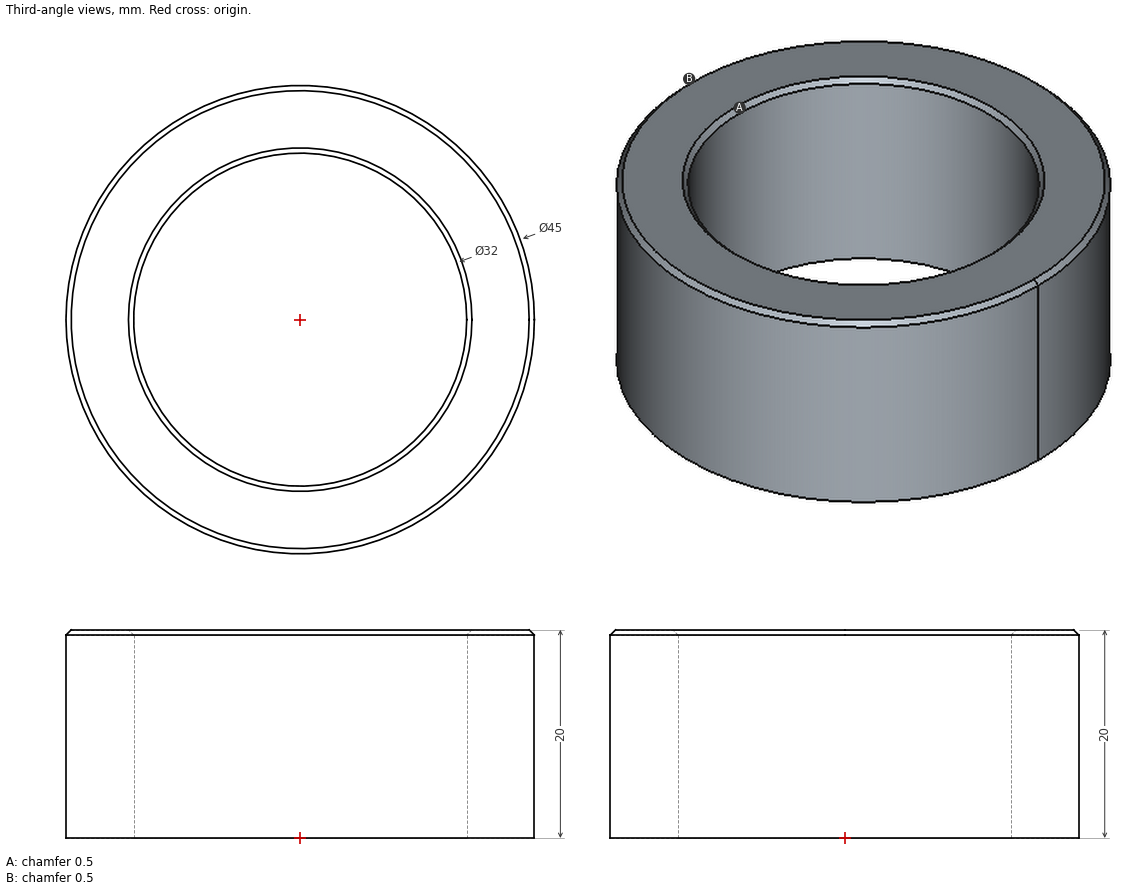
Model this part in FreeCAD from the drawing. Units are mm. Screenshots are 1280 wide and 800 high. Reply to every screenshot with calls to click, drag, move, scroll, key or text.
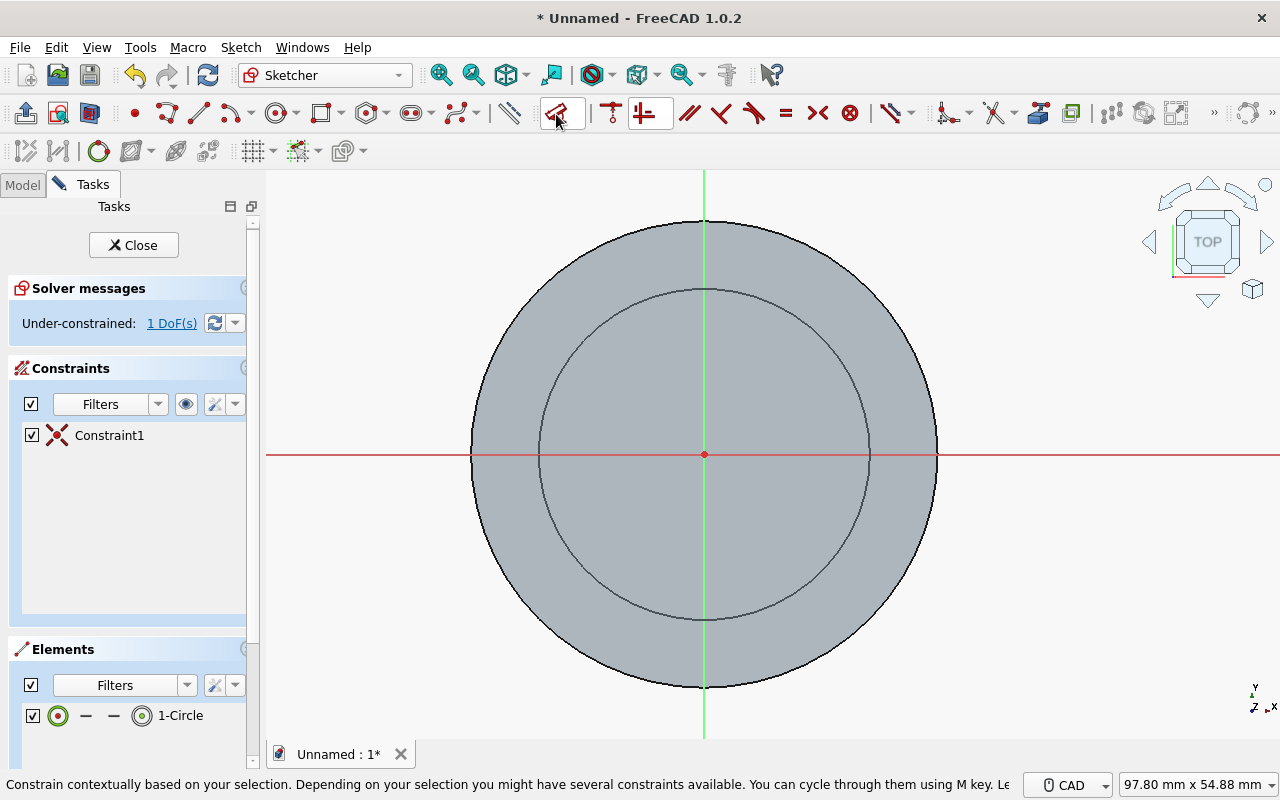
click(821, 337)
click(844, 314)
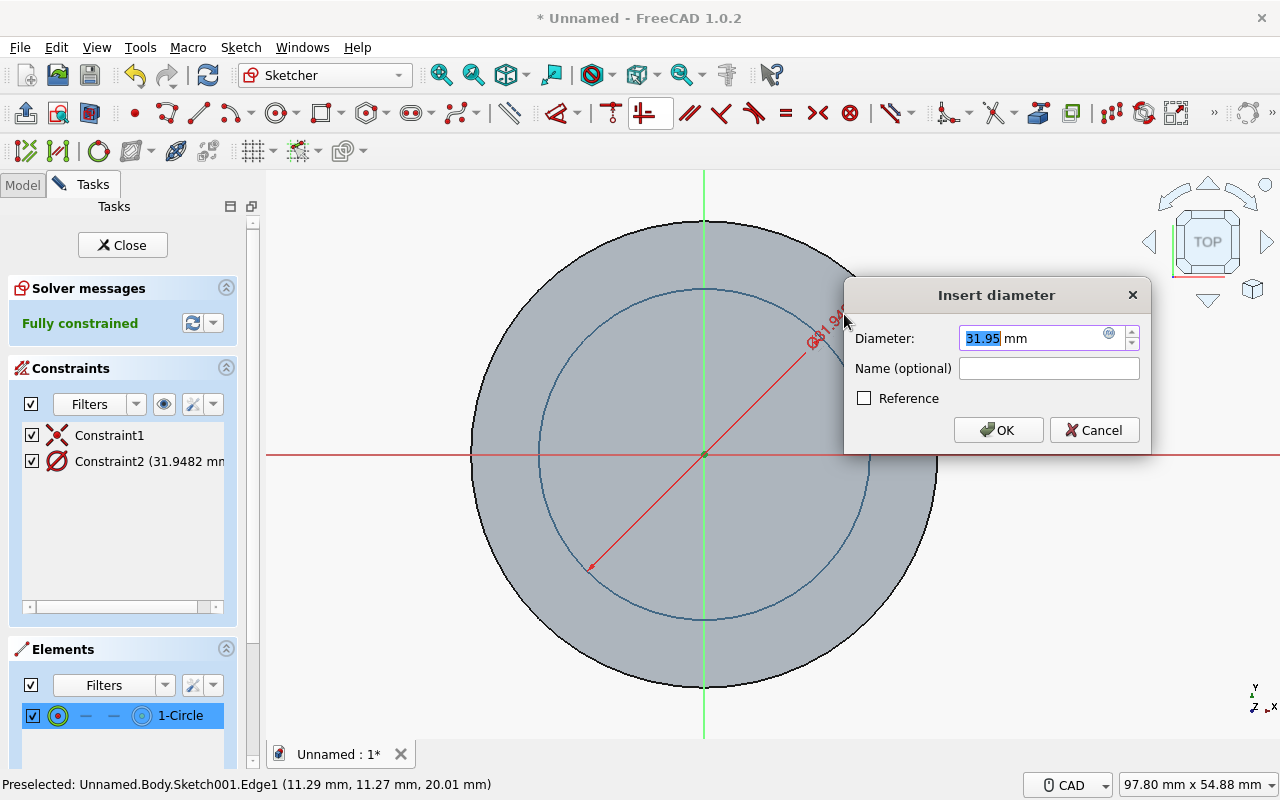
text(32)
key(Return)
key(Escape)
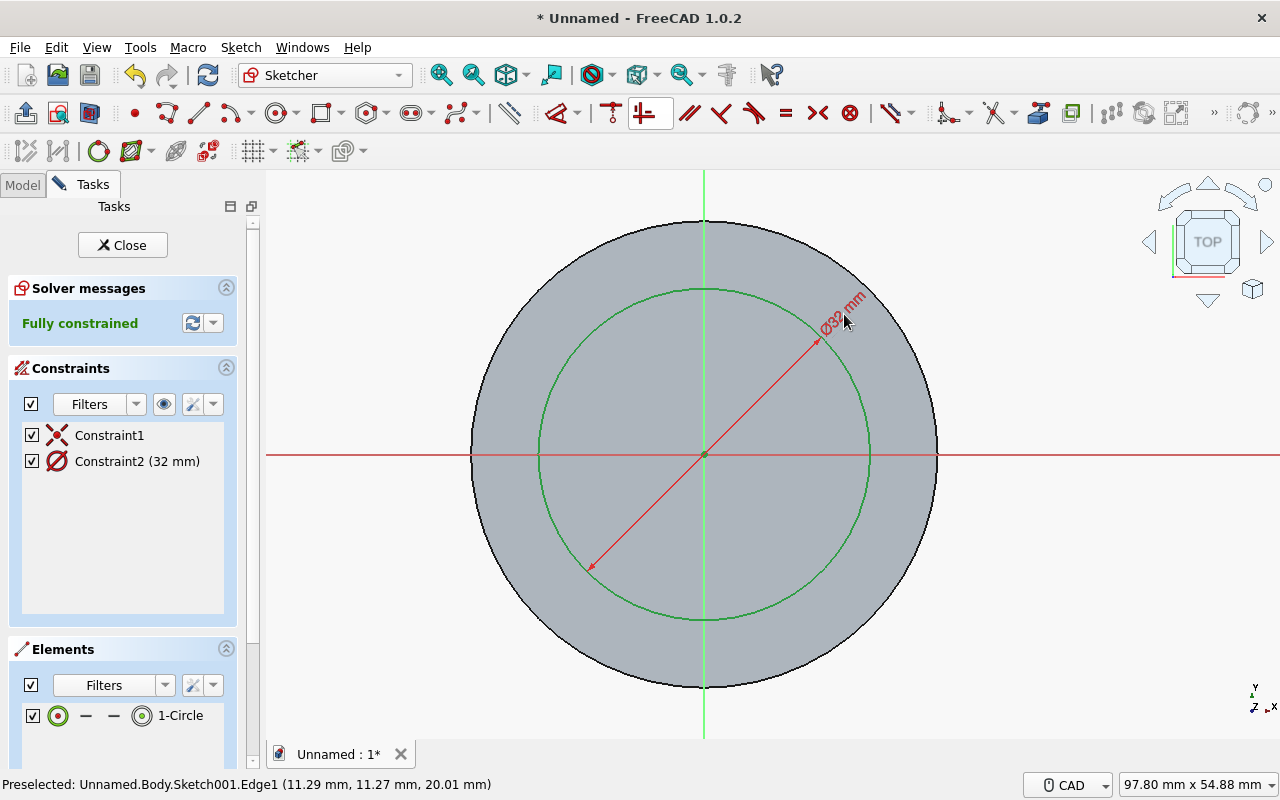
click(123, 245)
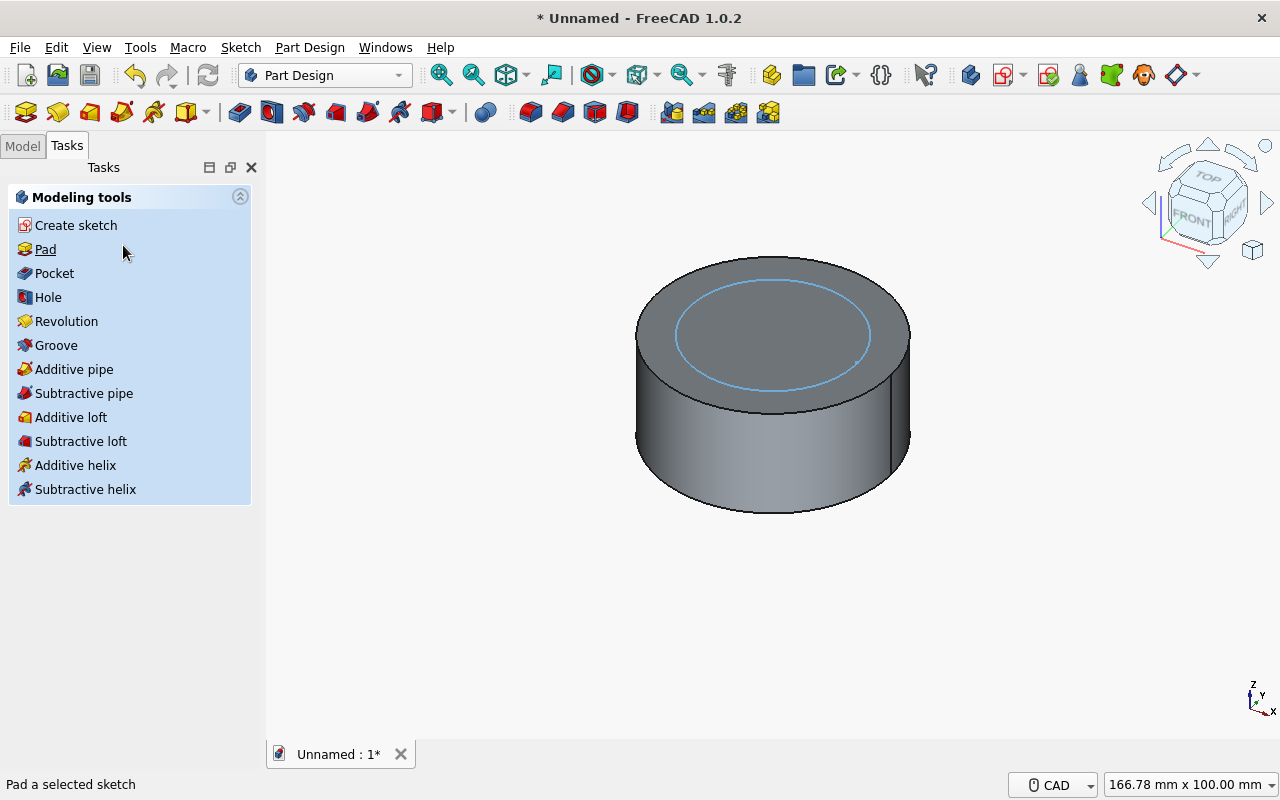
click(240, 112)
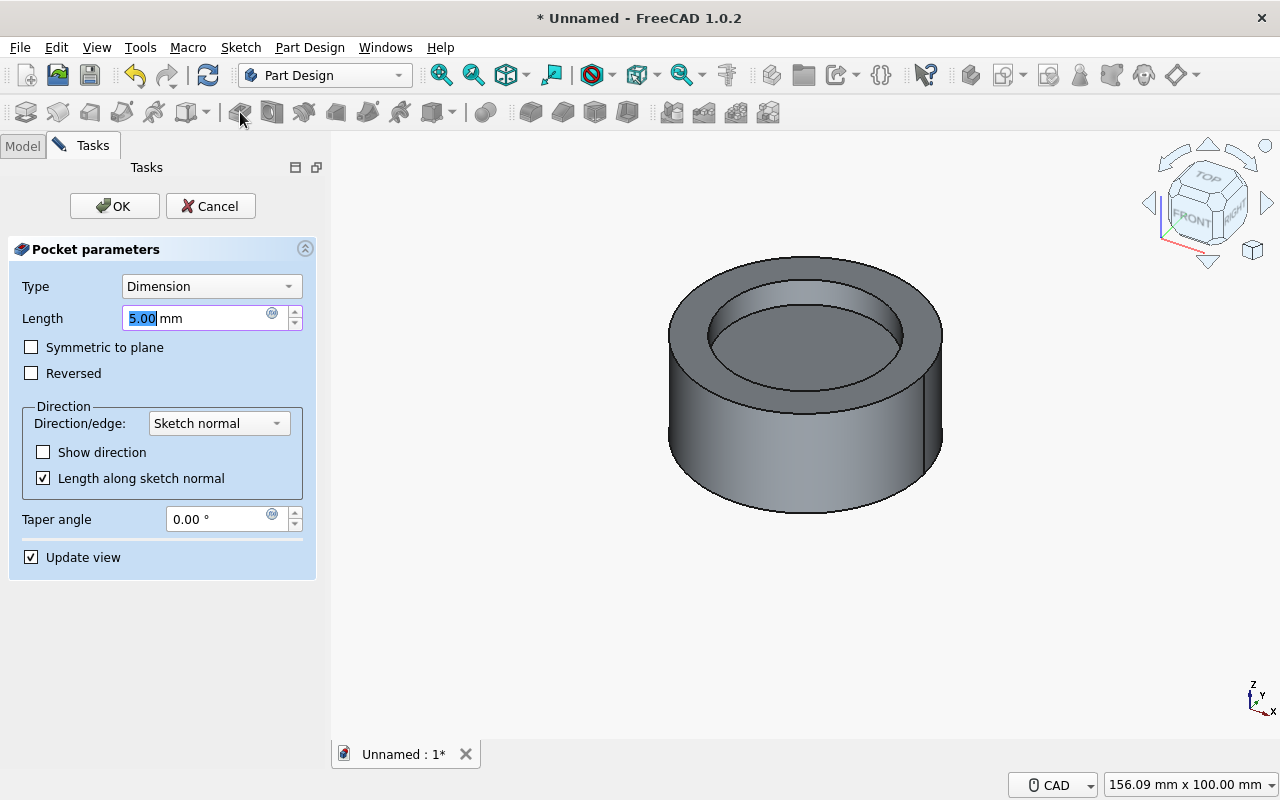
text(20)
key(Tab)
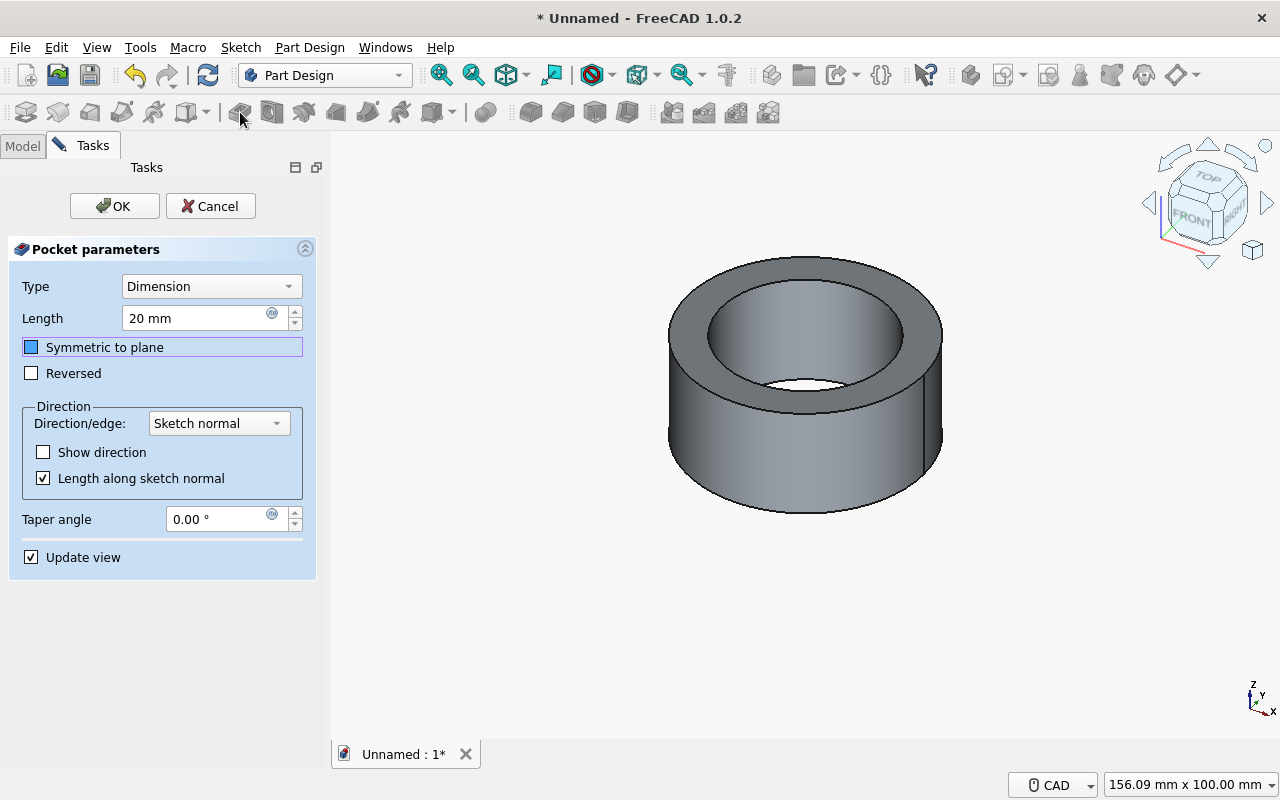
click(115, 206)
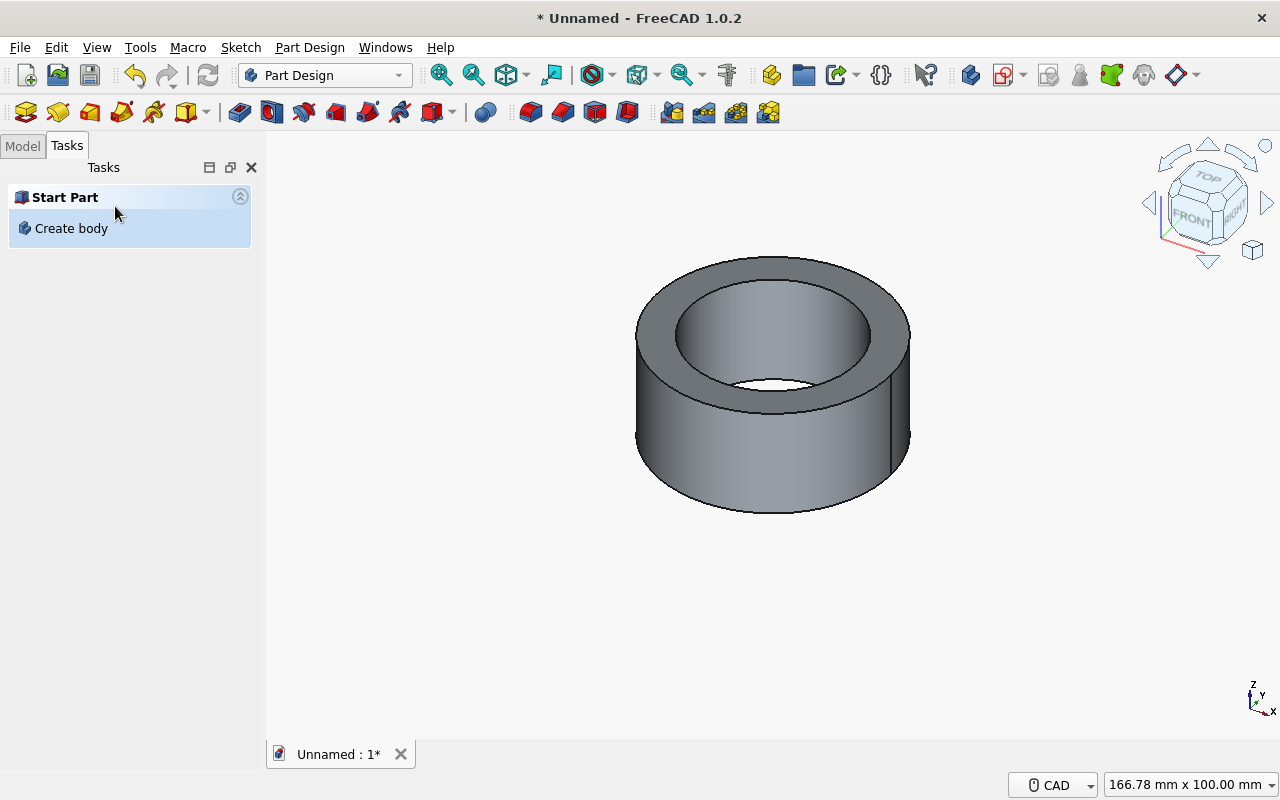
click(689, 306)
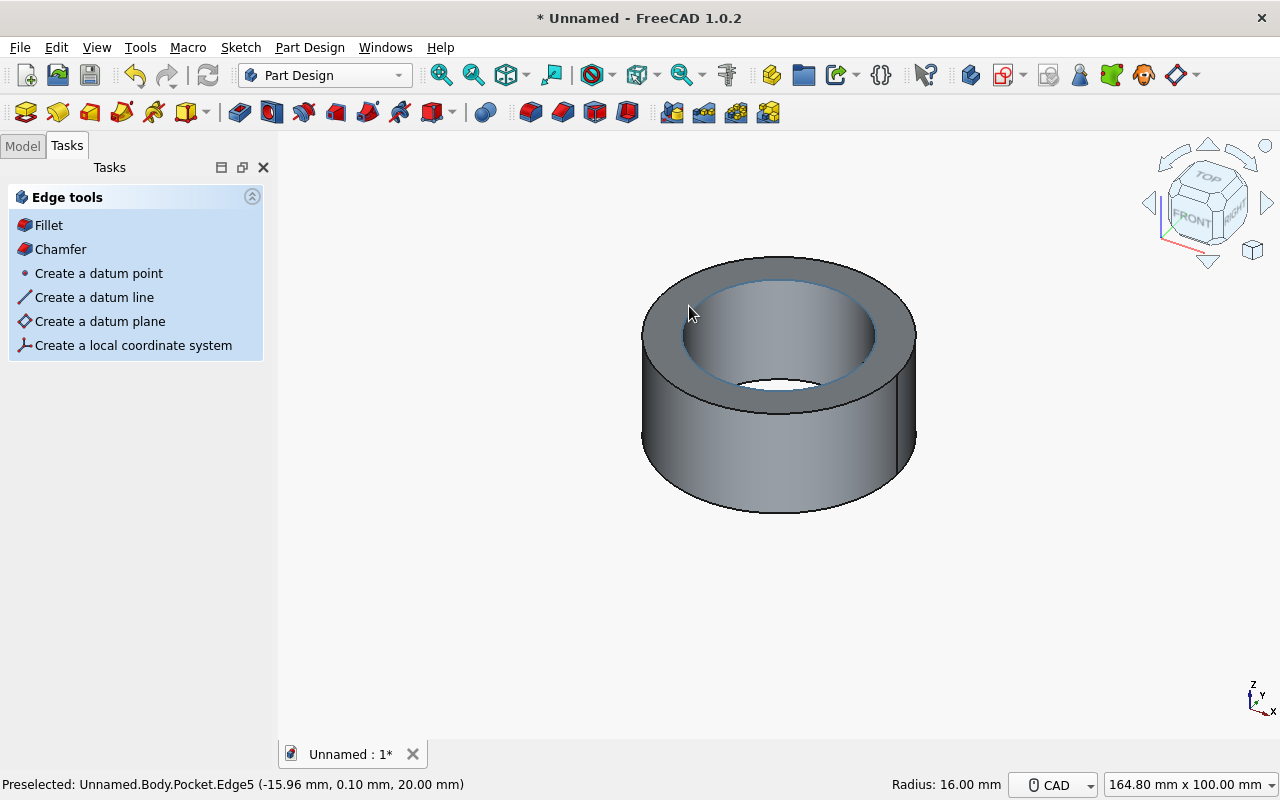
click(564, 112)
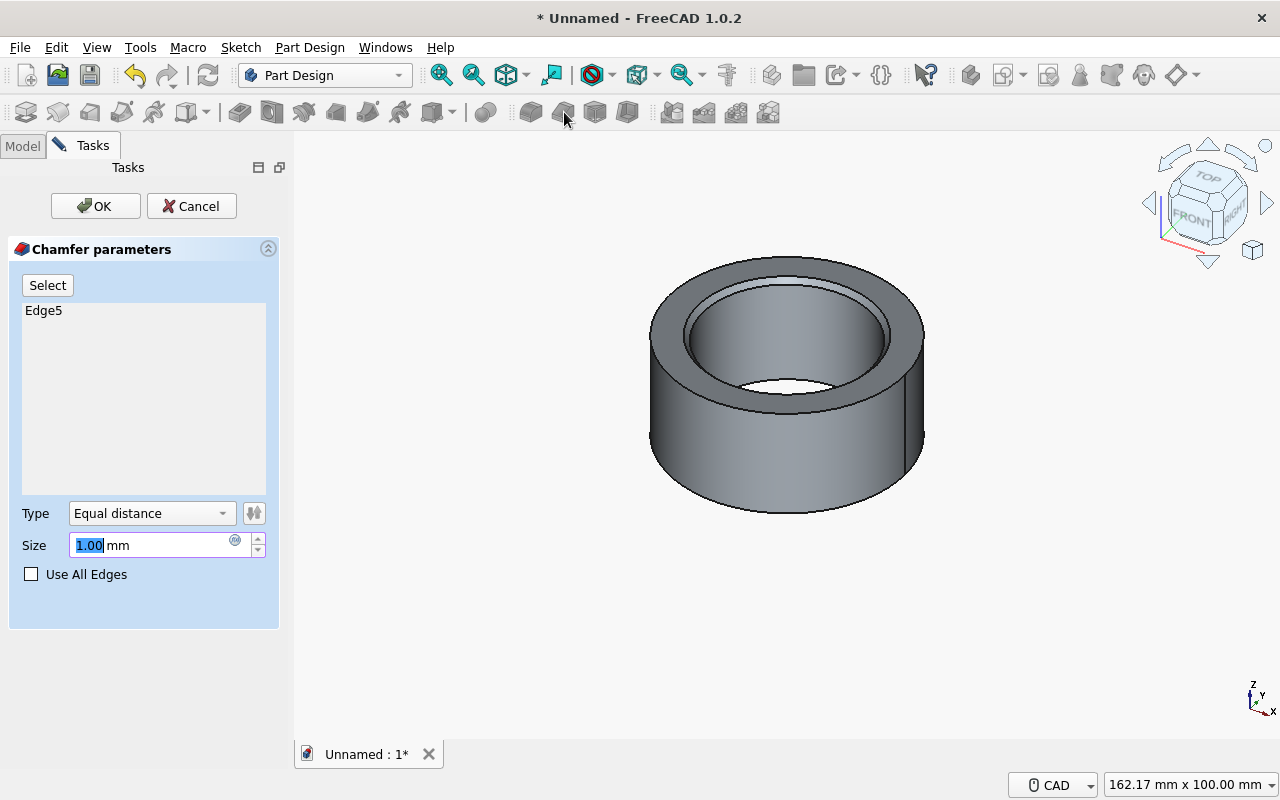
text(0.5)
key(Tab)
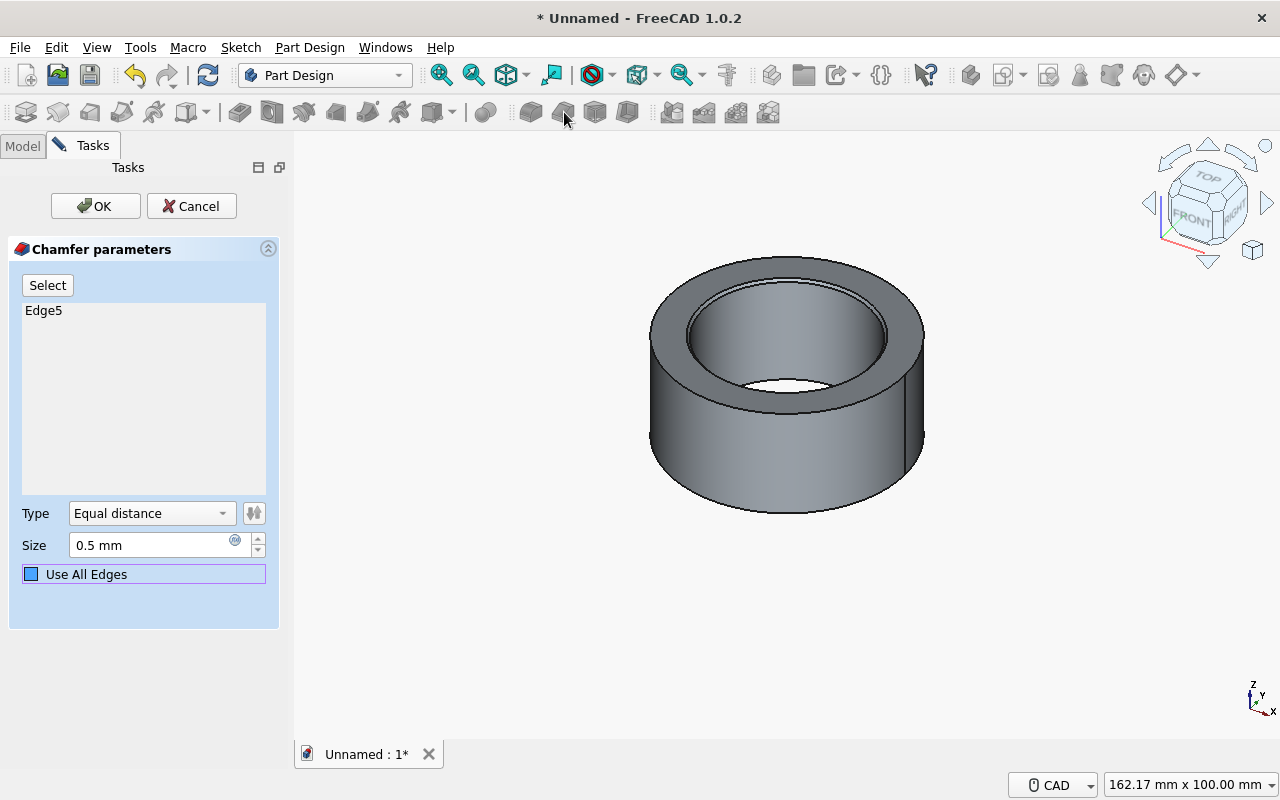
click(96, 206)